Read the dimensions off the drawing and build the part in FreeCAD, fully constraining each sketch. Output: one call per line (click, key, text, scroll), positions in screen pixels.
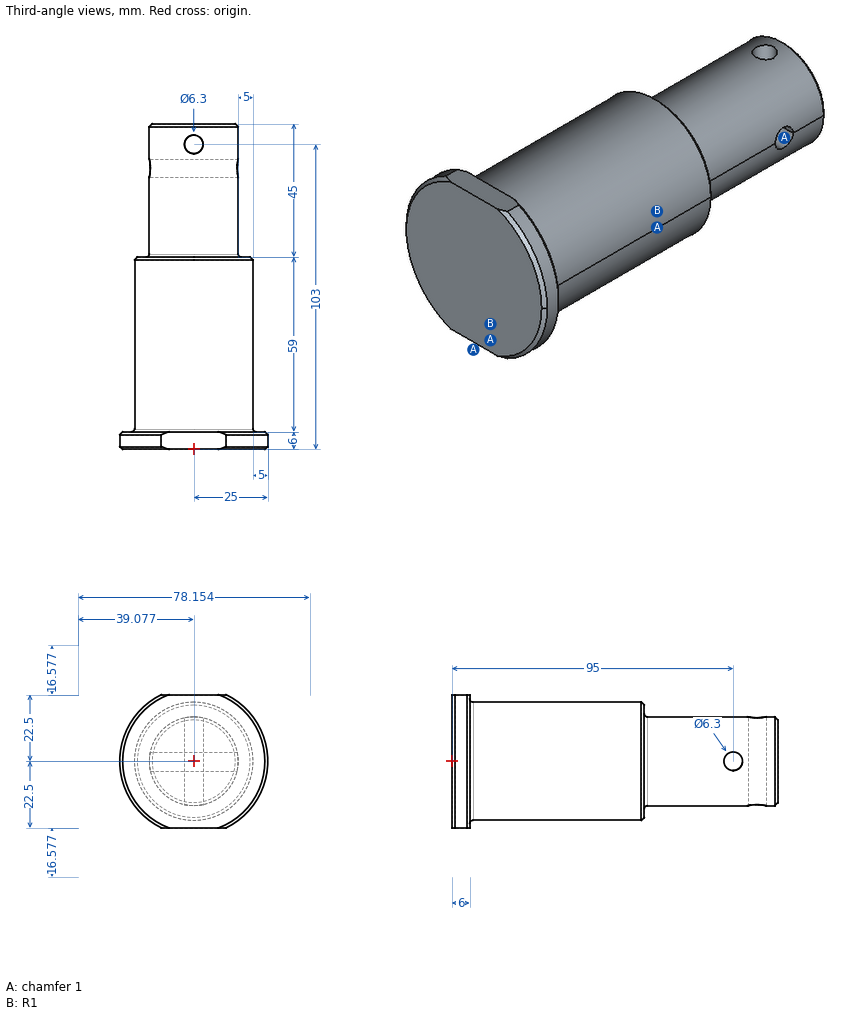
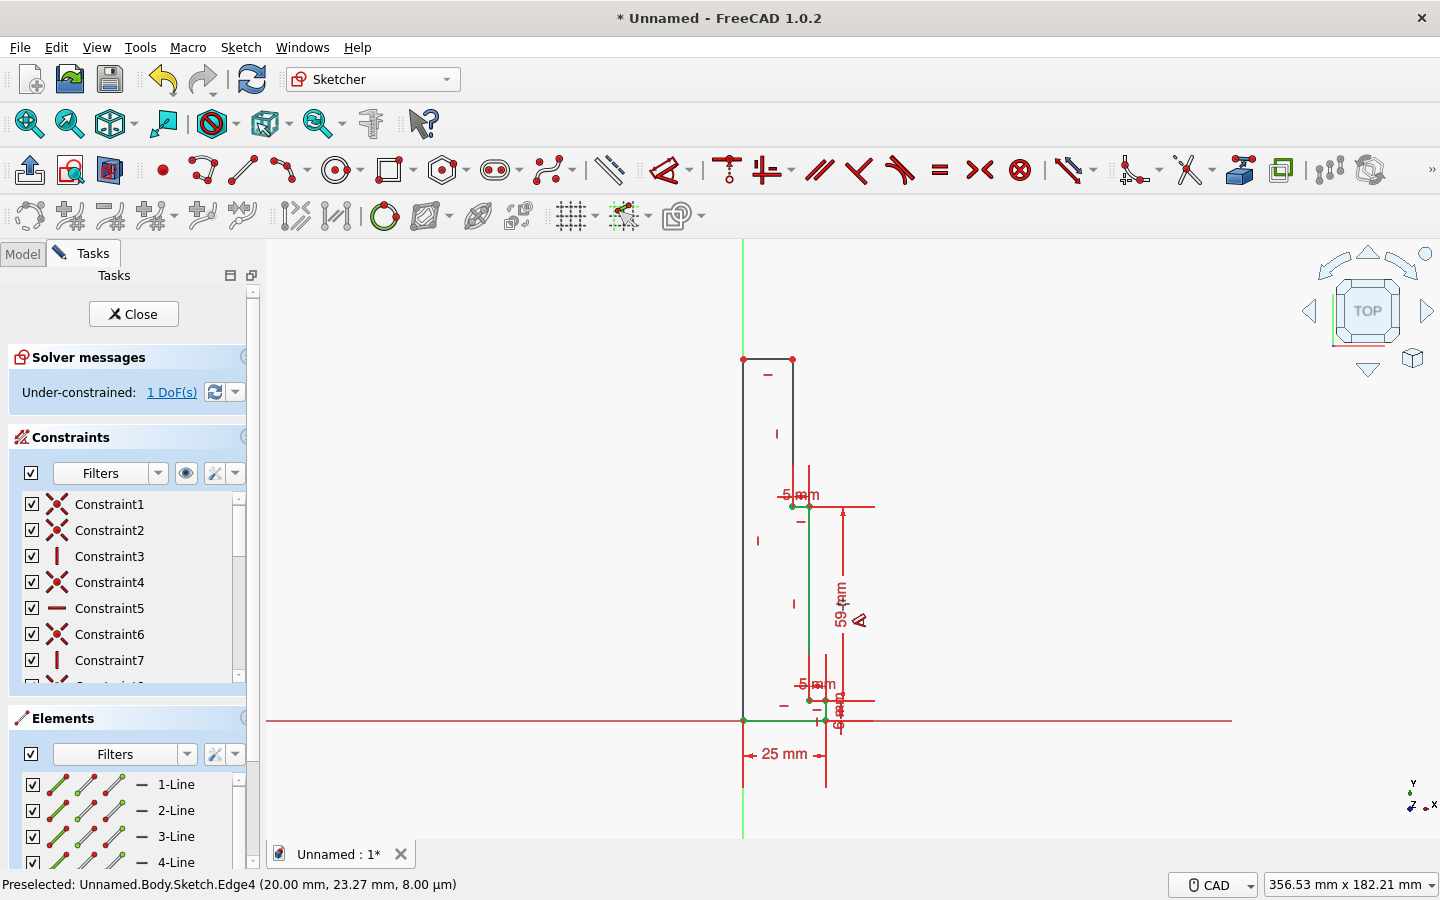
click(793, 462)
click(827, 433)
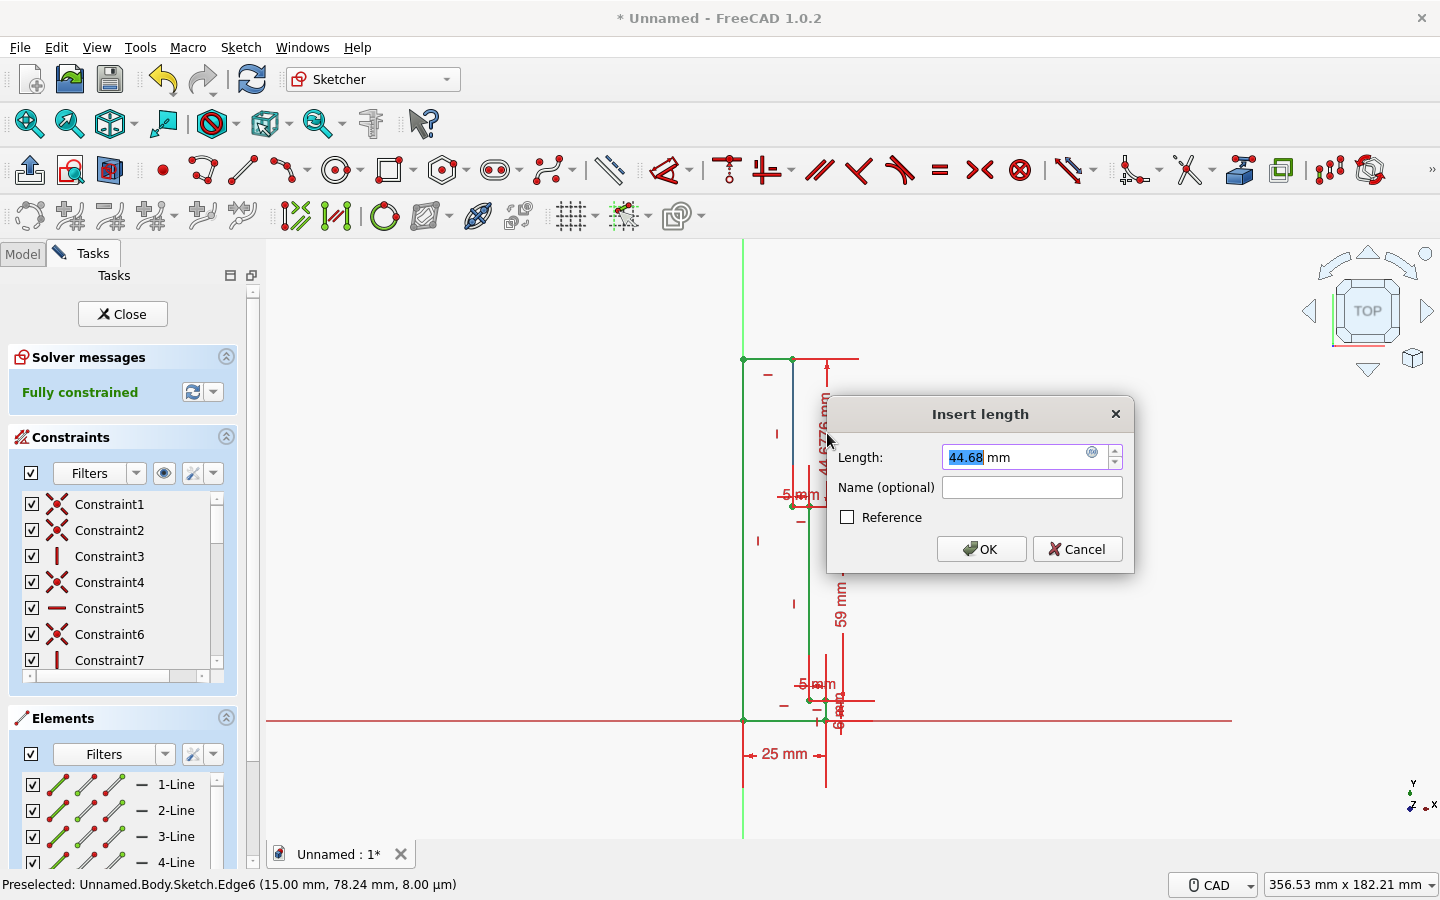
text(45)
key(Return)
key(Escape)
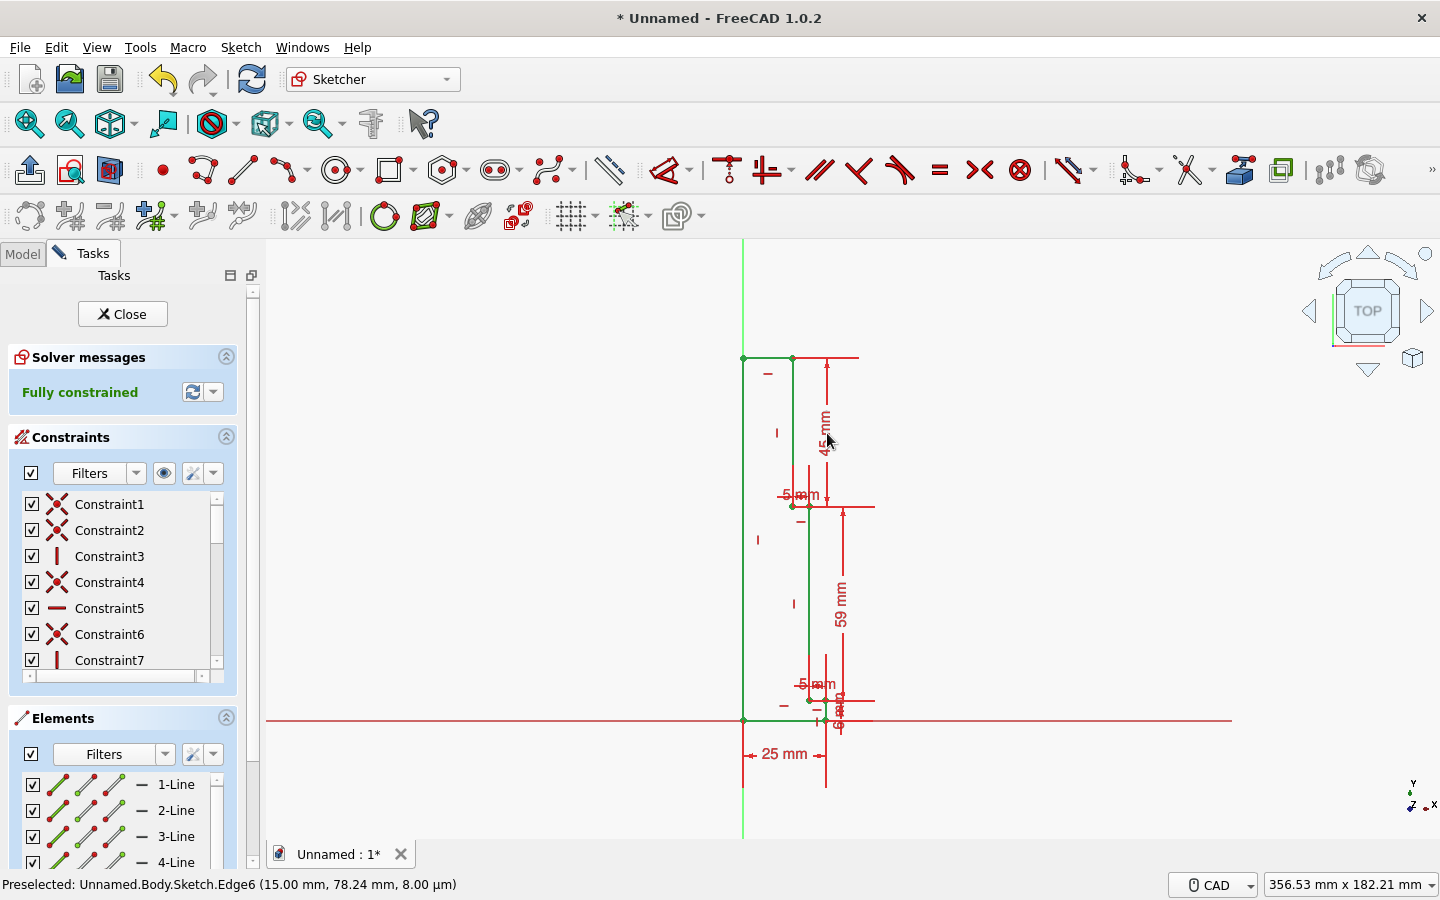
click(123, 314)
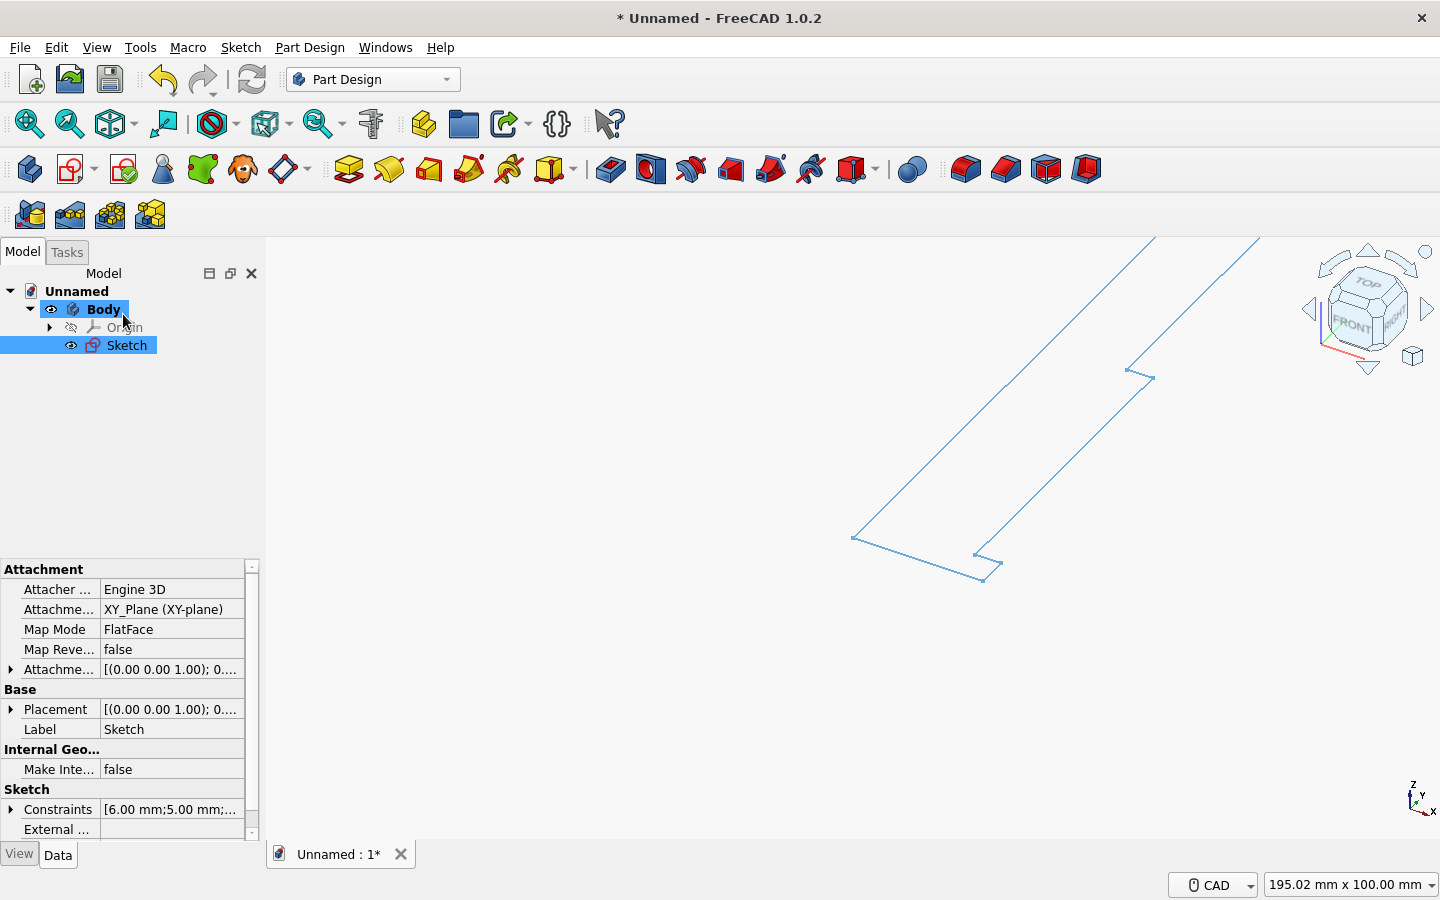
click(390, 170)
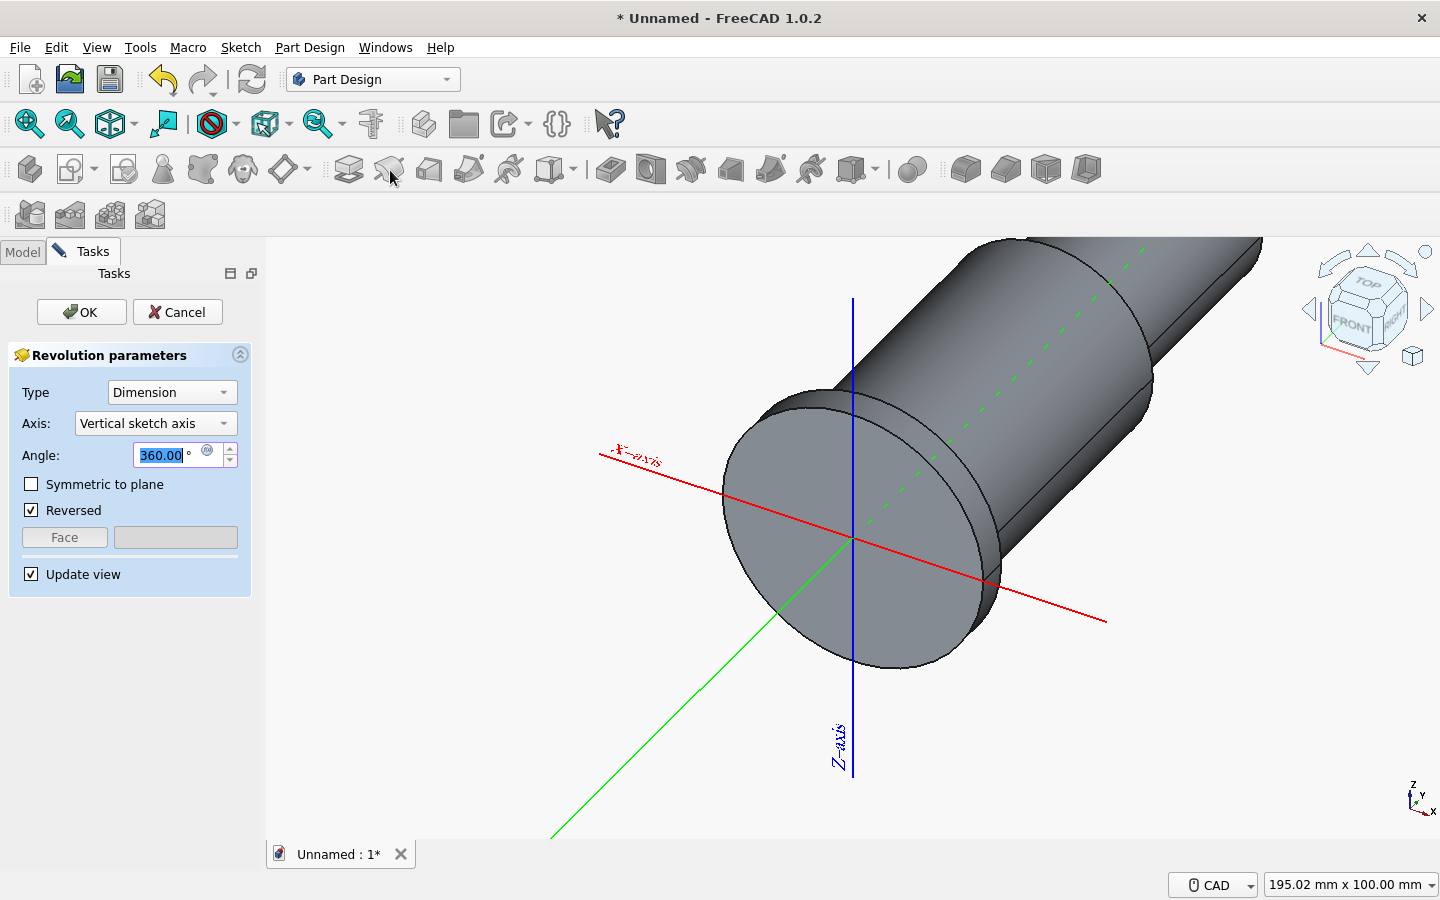
click(82, 312)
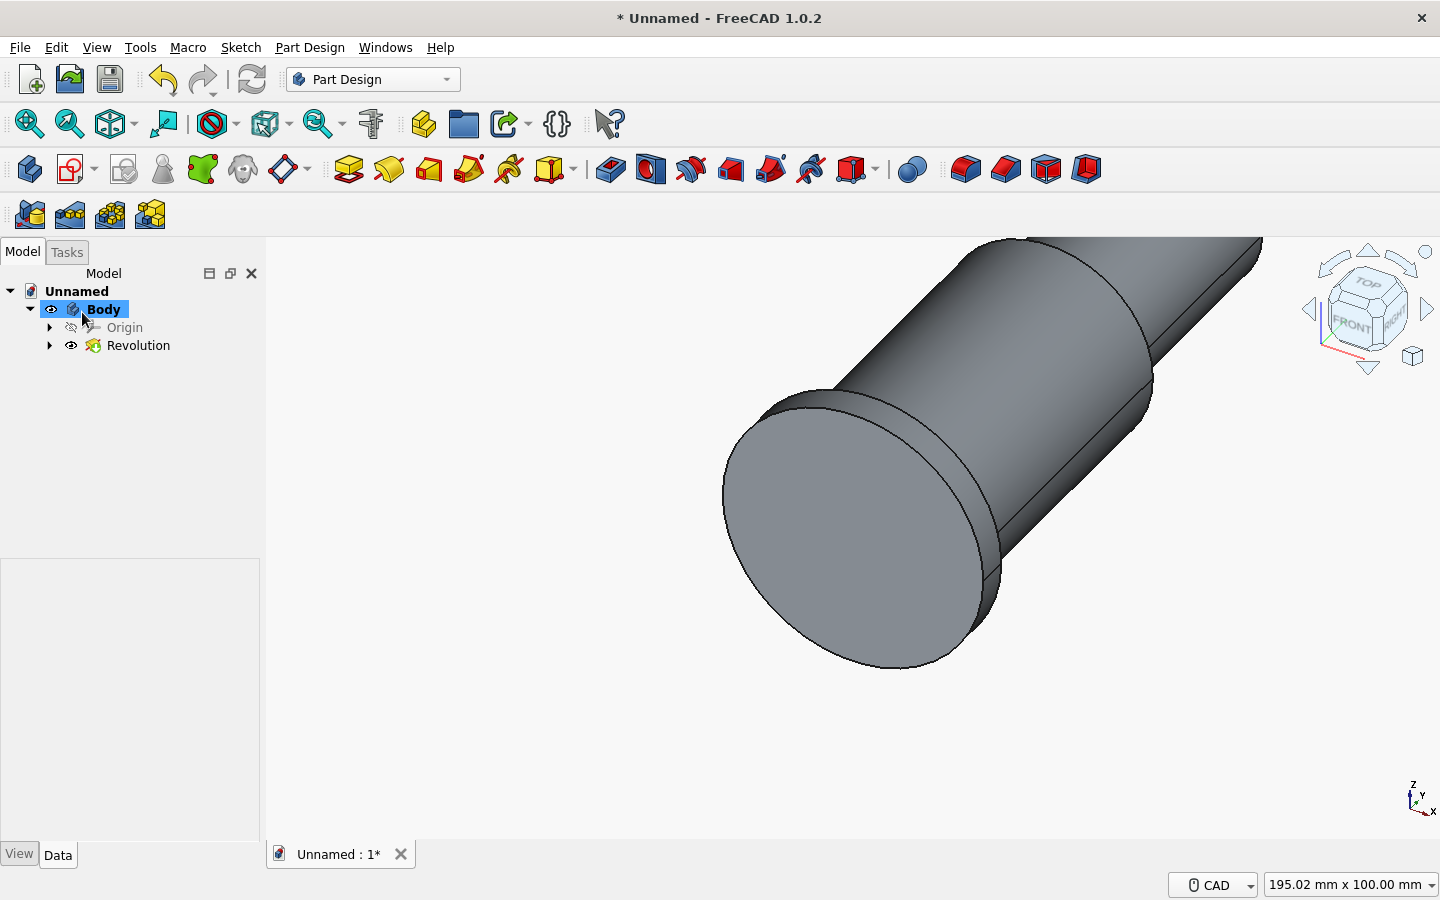
key(v)
key(f)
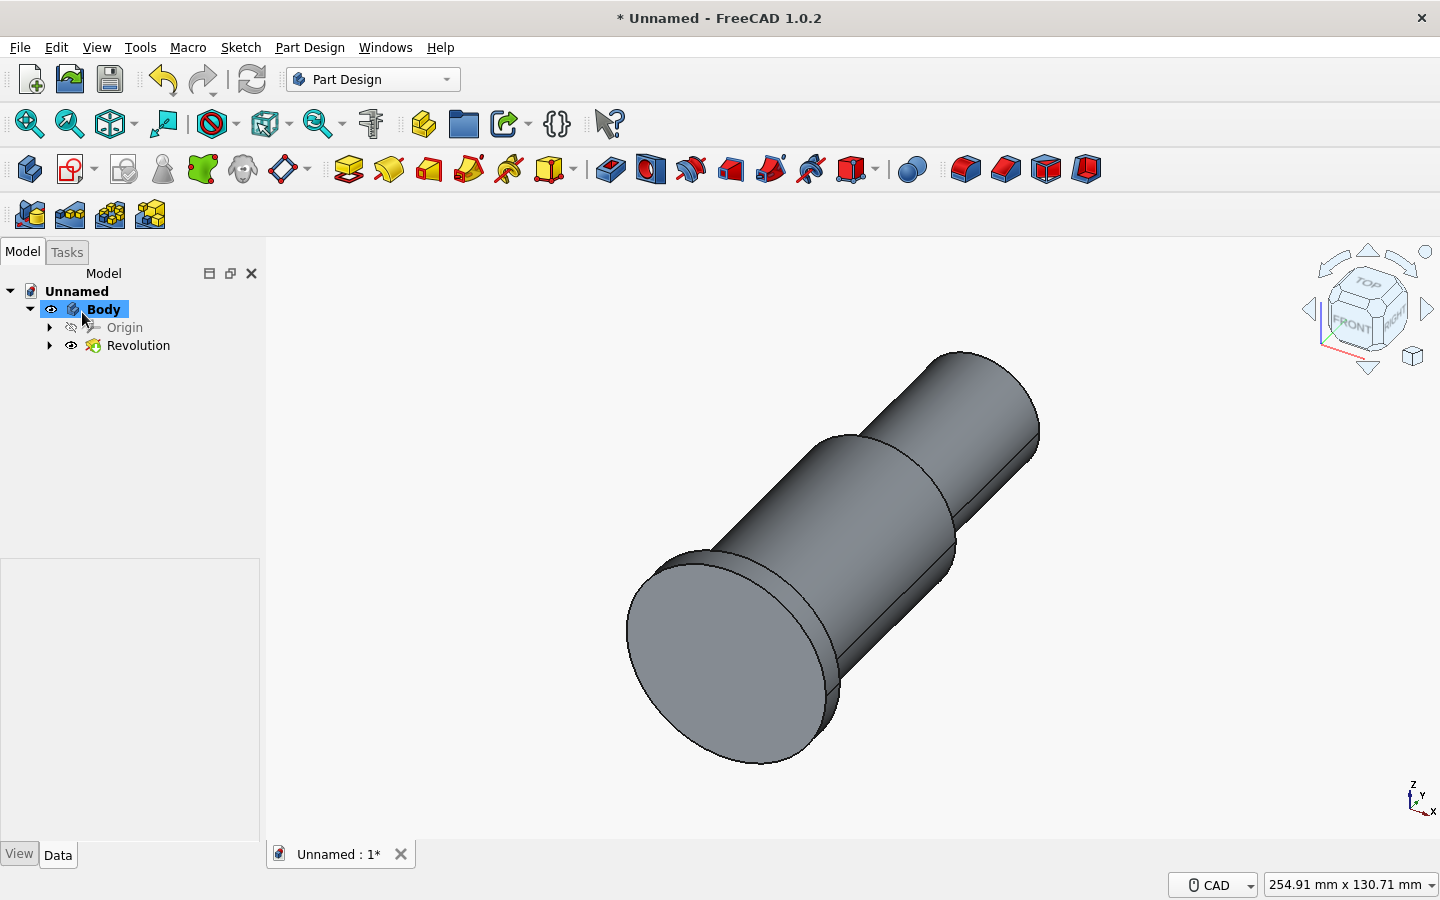
click(646, 581)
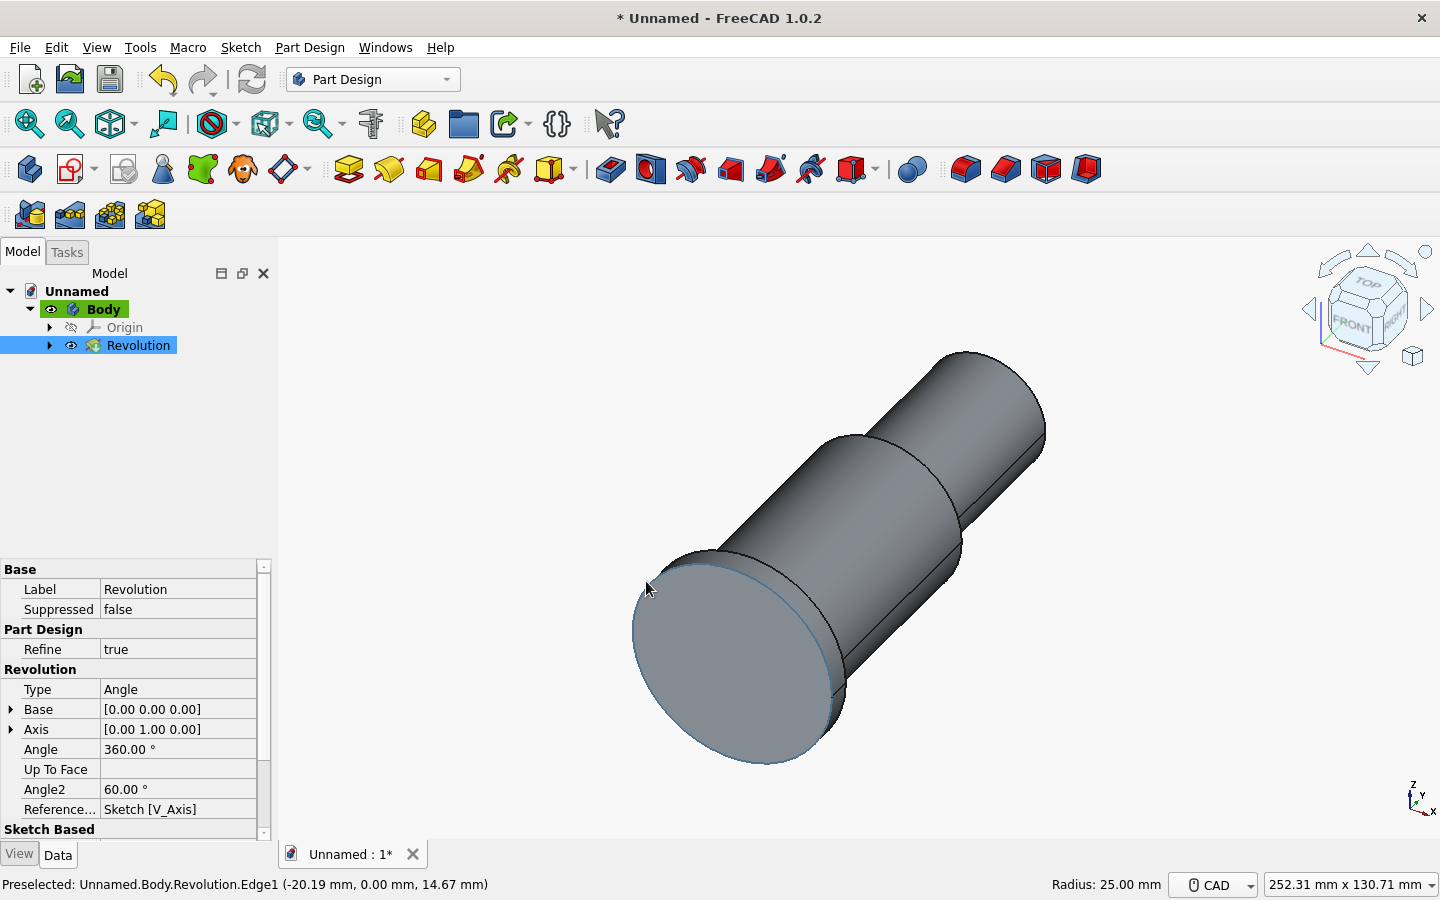
key(0)